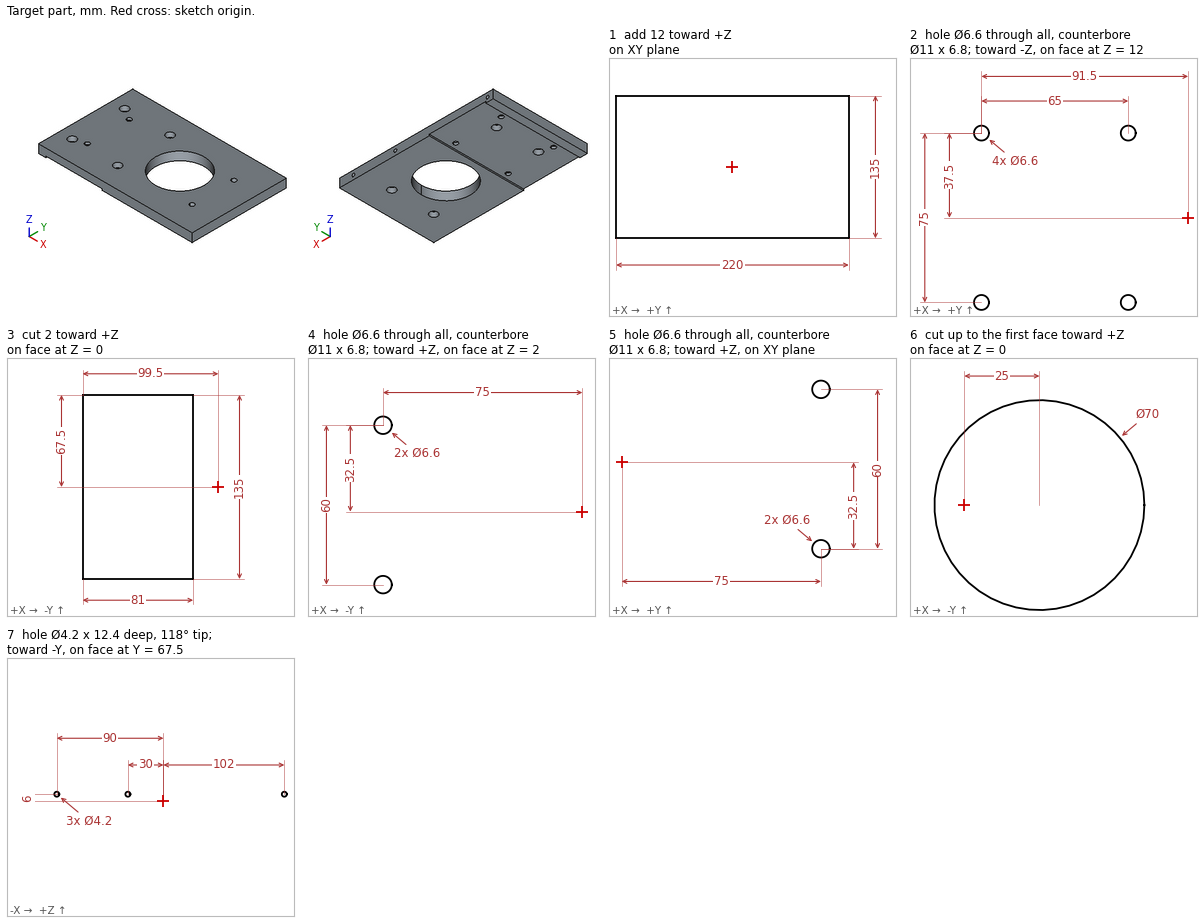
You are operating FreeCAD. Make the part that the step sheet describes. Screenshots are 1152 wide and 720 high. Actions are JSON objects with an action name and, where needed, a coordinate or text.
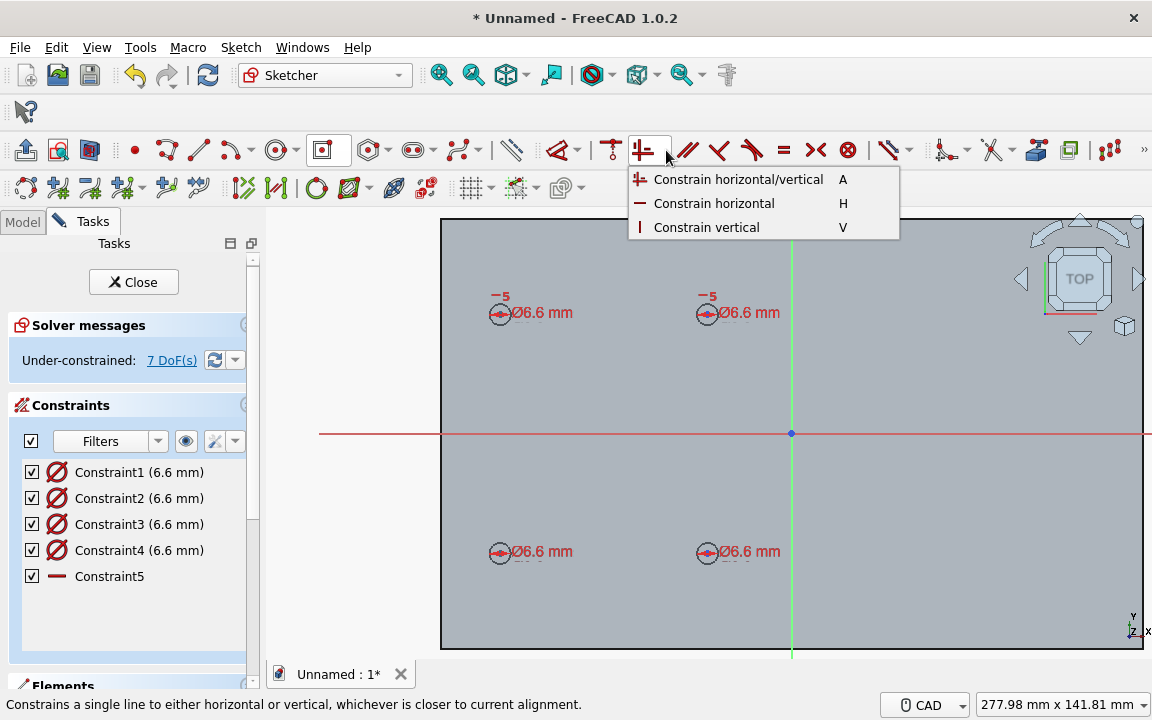
{"action": "left_click", "coordinate": [764, 227]}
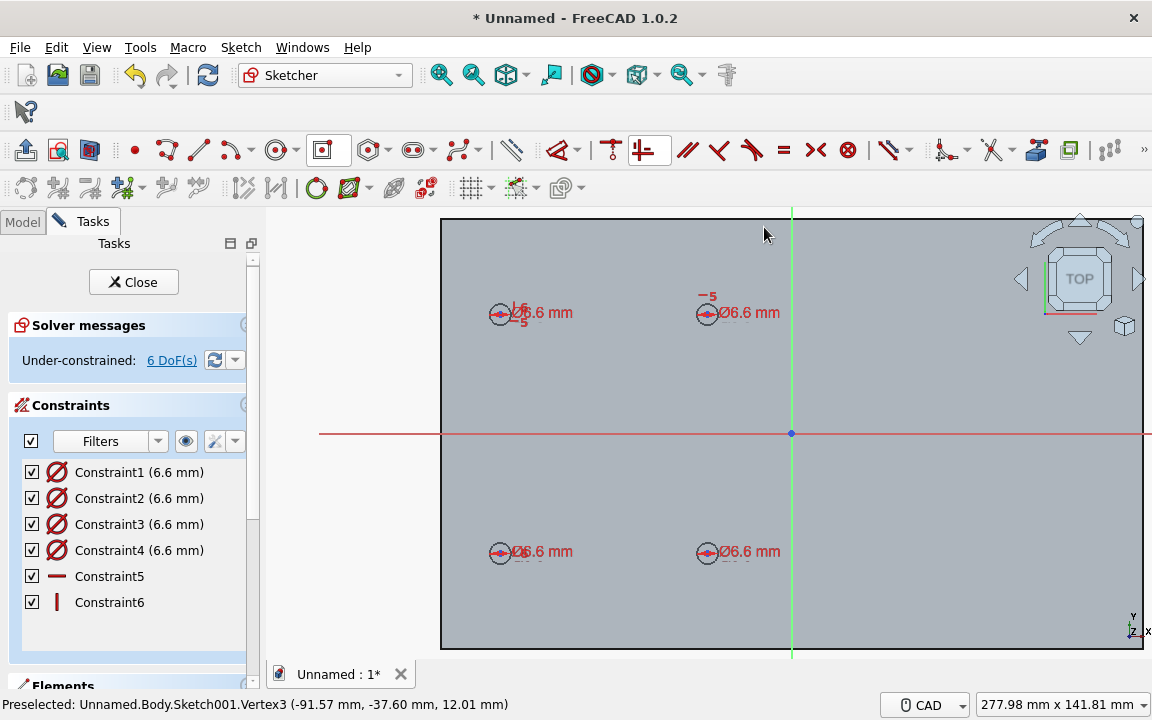
{"action": "left_click", "coordinate": [707, 315]}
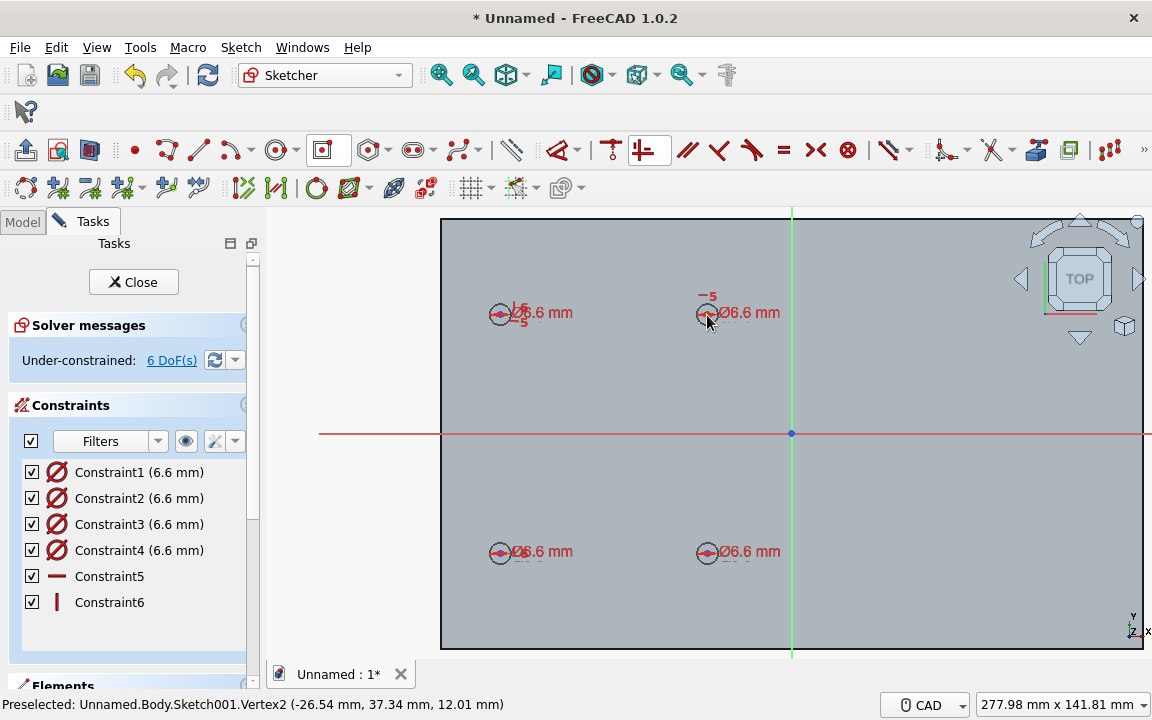
{"action": "left_click", "coordinate": [708, 554]}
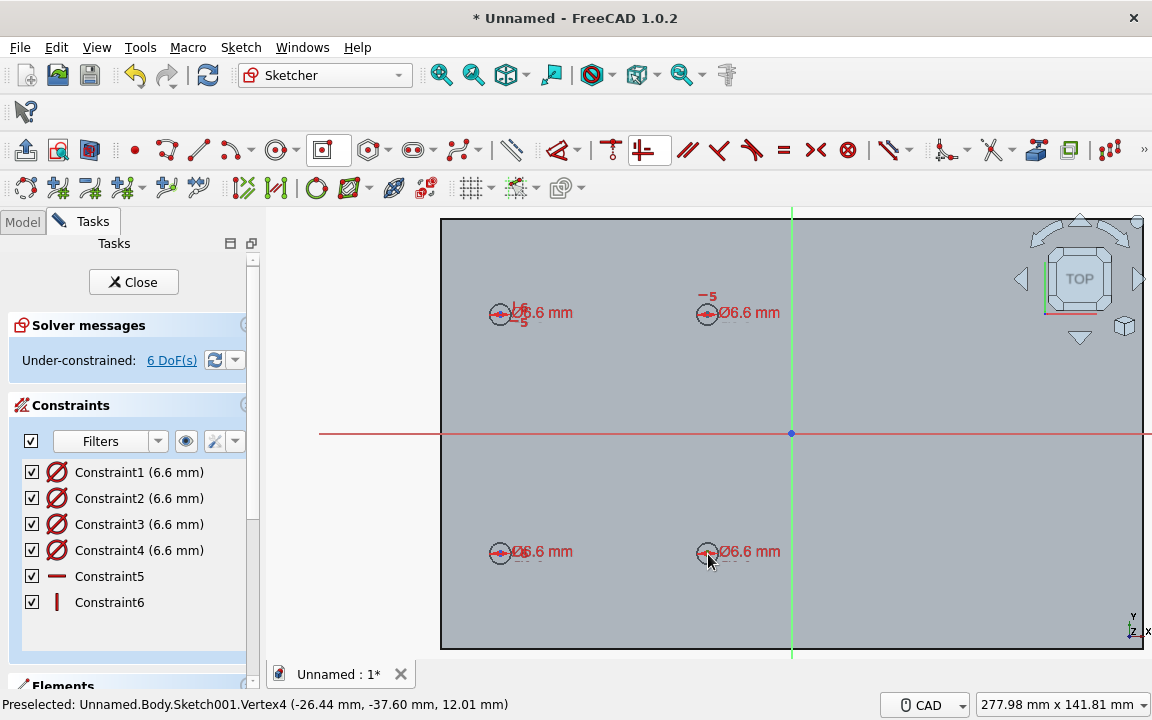
{"action": "key", "text": "v"}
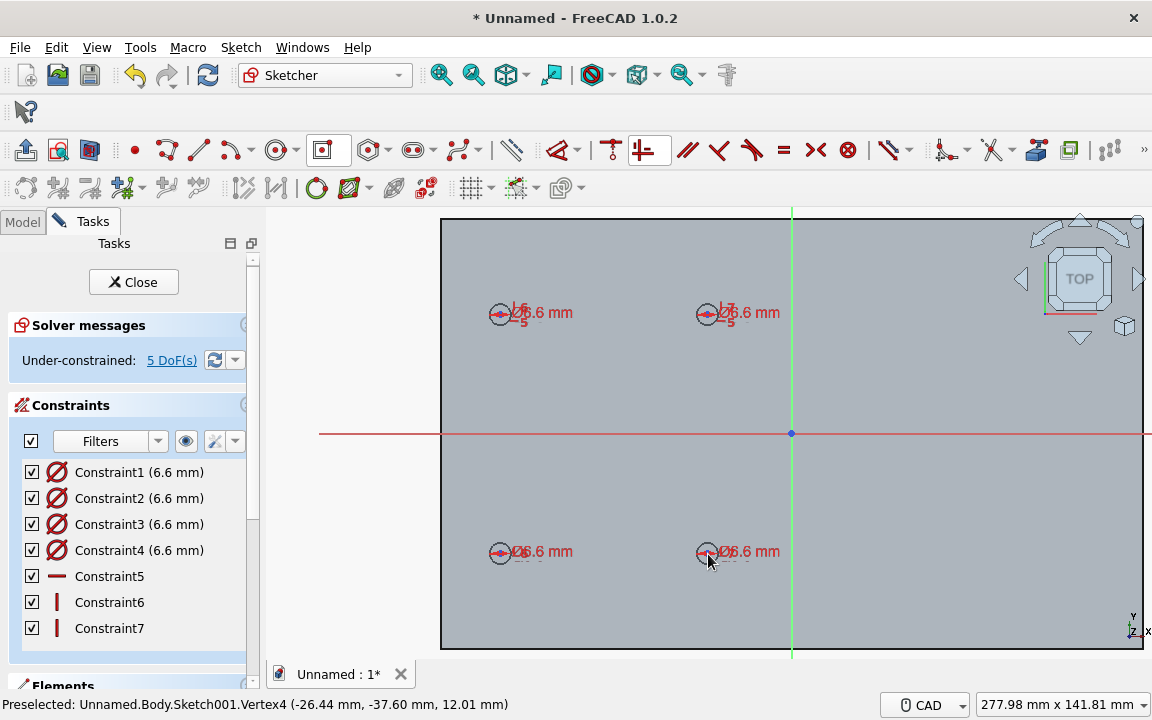
{"action": "left_click", "coordinate": [500, 554]}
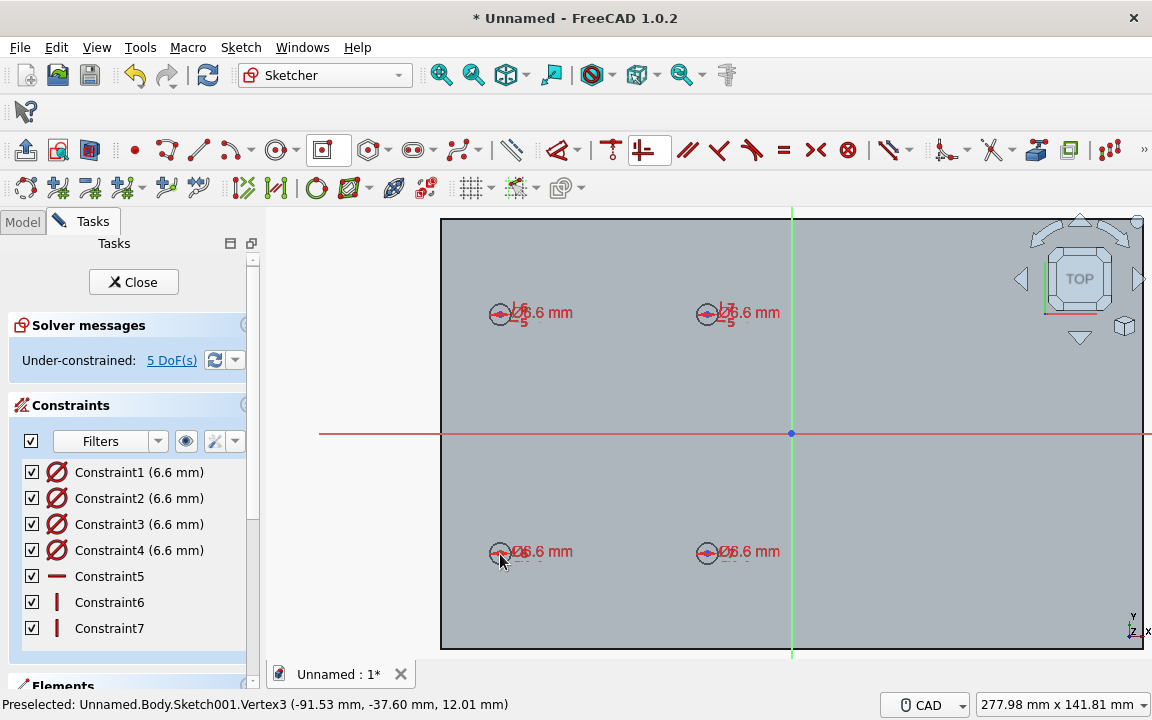
{"action": "left_click", "coordinate": [707, 554]}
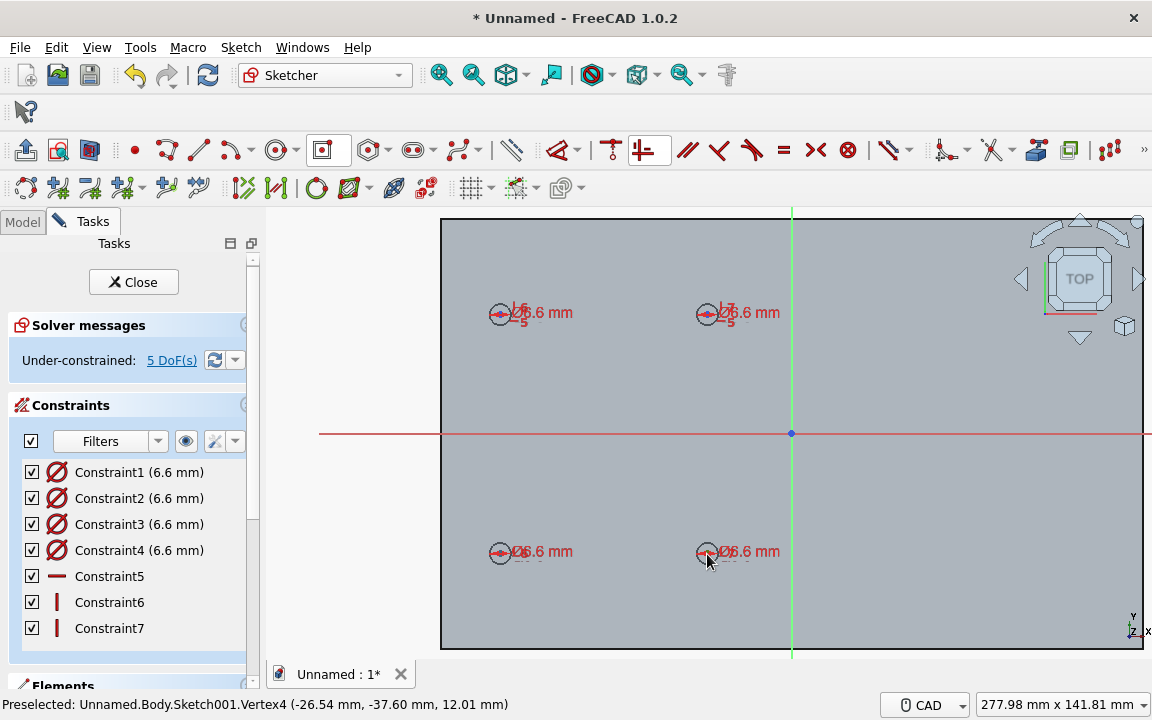
{"action": "key", "text": "h"}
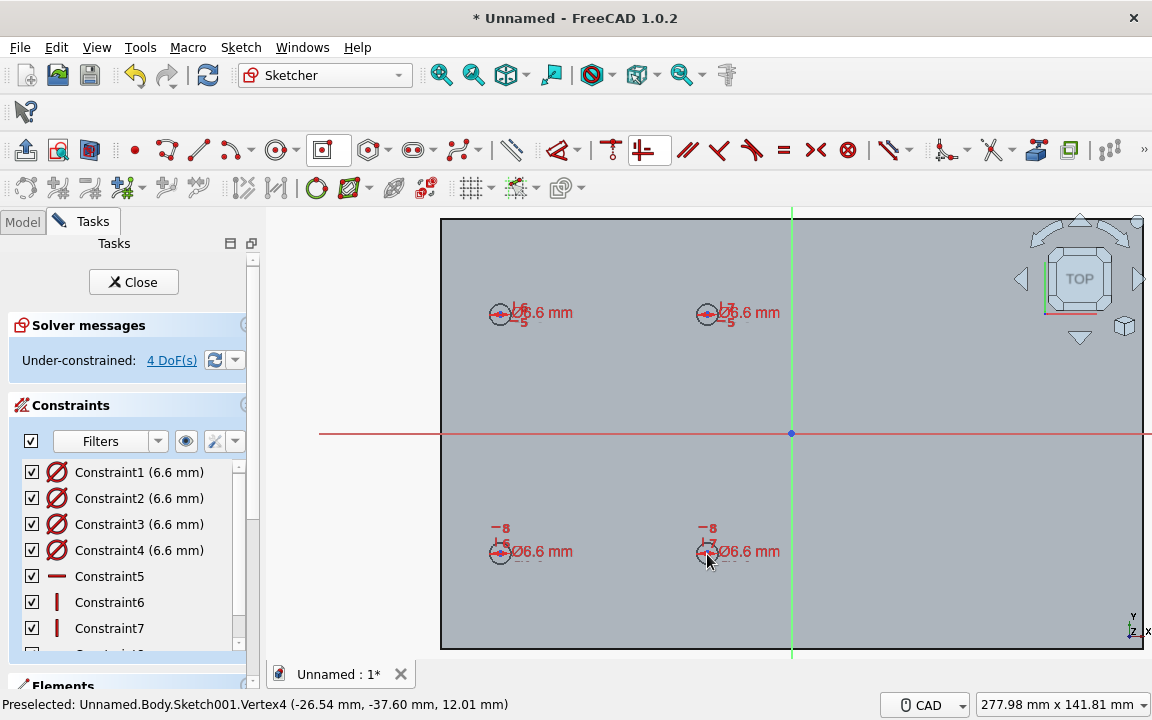
{"action": "left_click", "coordinate": [558, 150]}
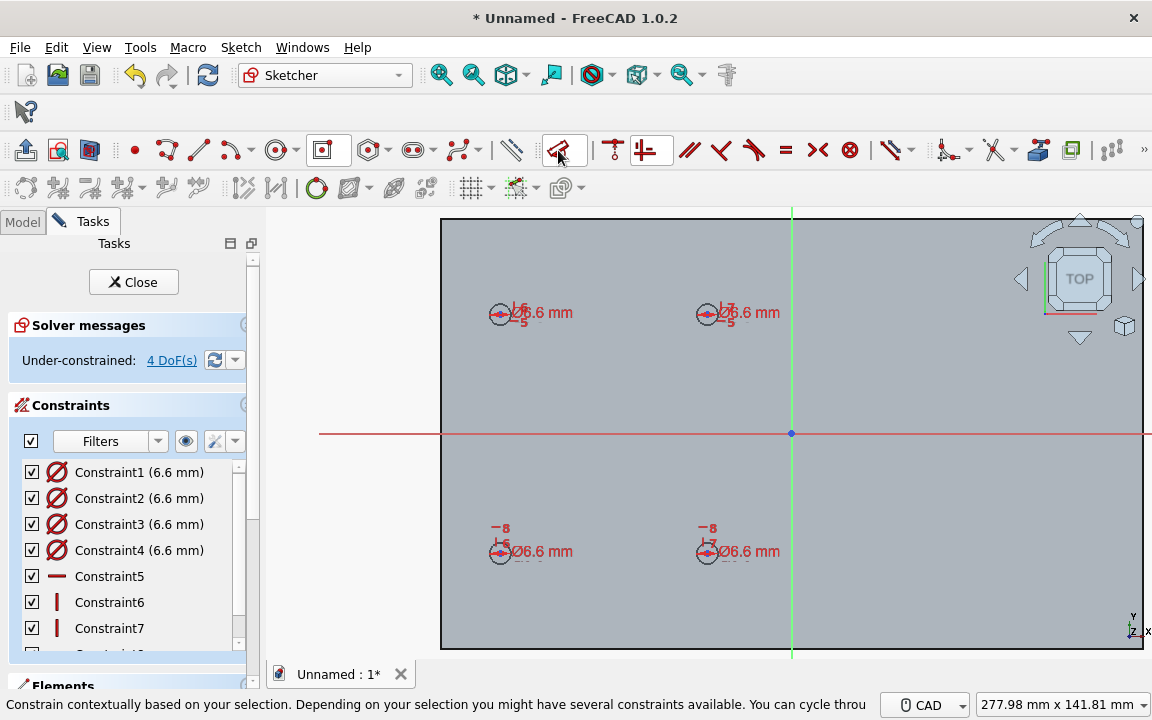
{"action": "left_click", "coordinate": [500, 315]}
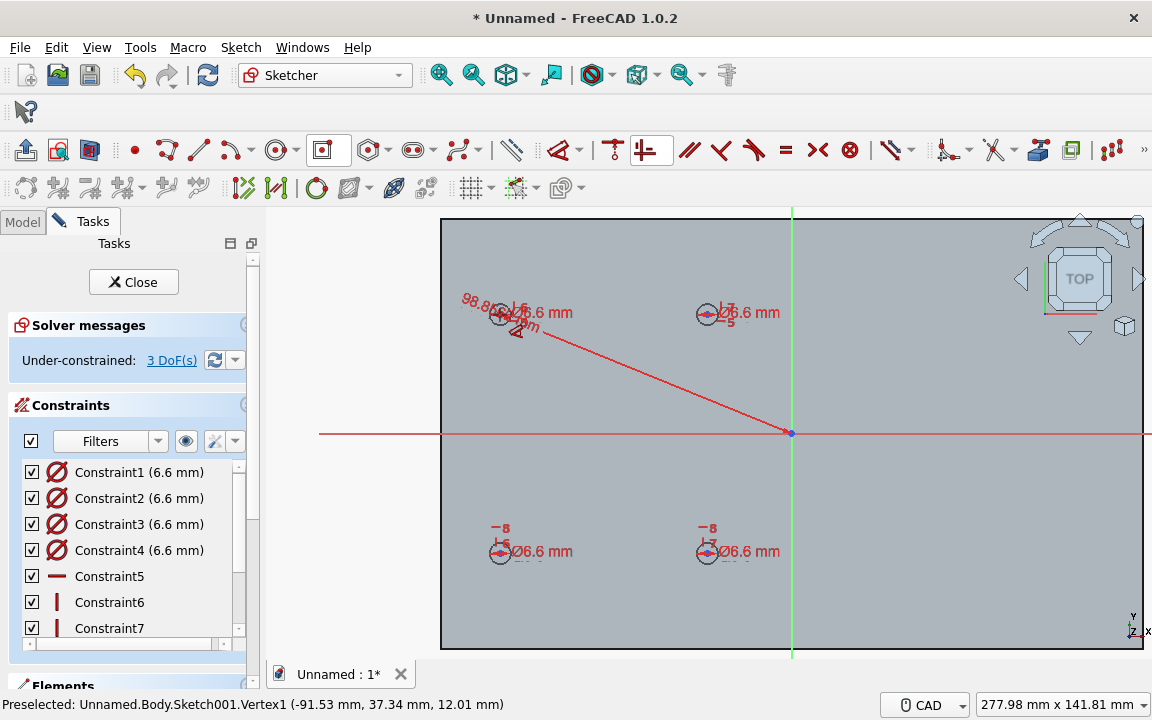
{"action": "left_click", "coordinate": [707, 315]}
{"action": "left_click", "coordinate": [604, 281]}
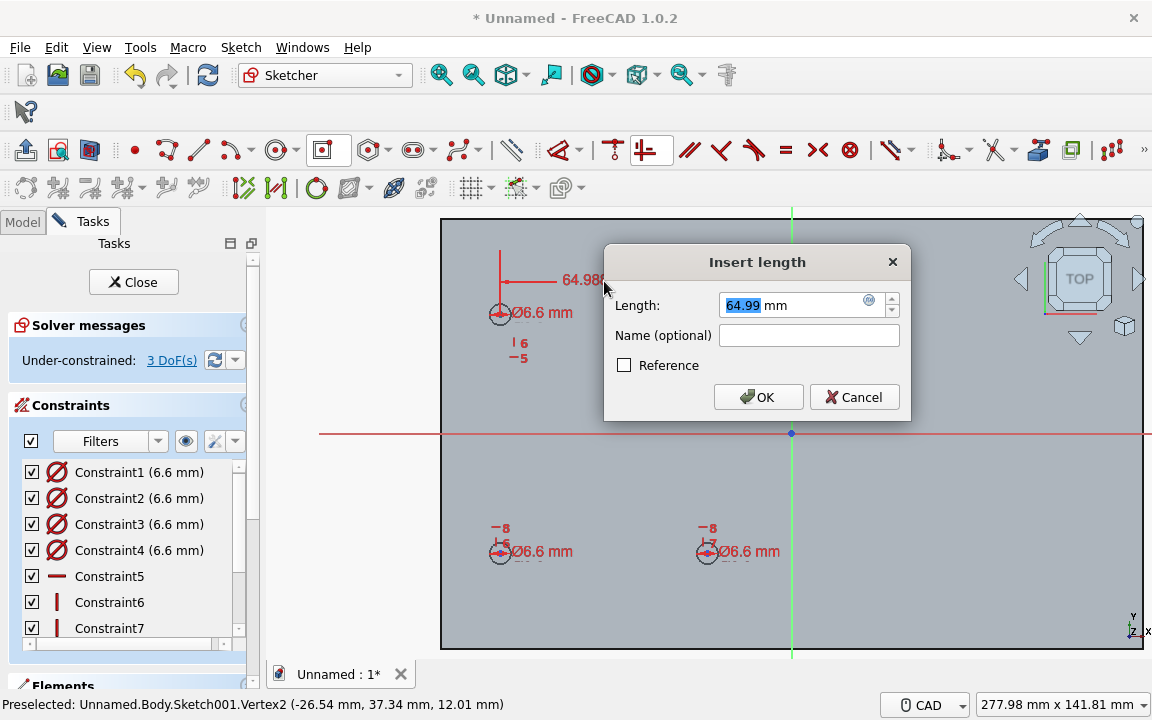
{"action": "type", "text": "65"}
{"action": "key", "text": "Return"}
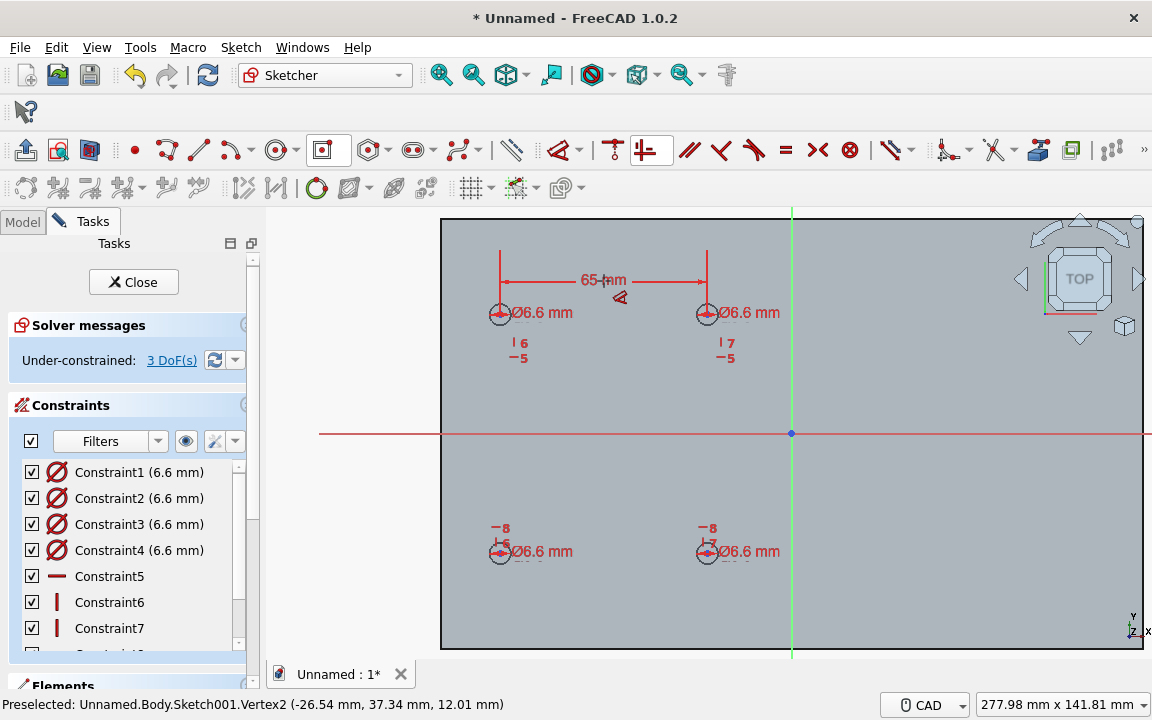
{"action": "left_click", "coordinate": [500, 315]}